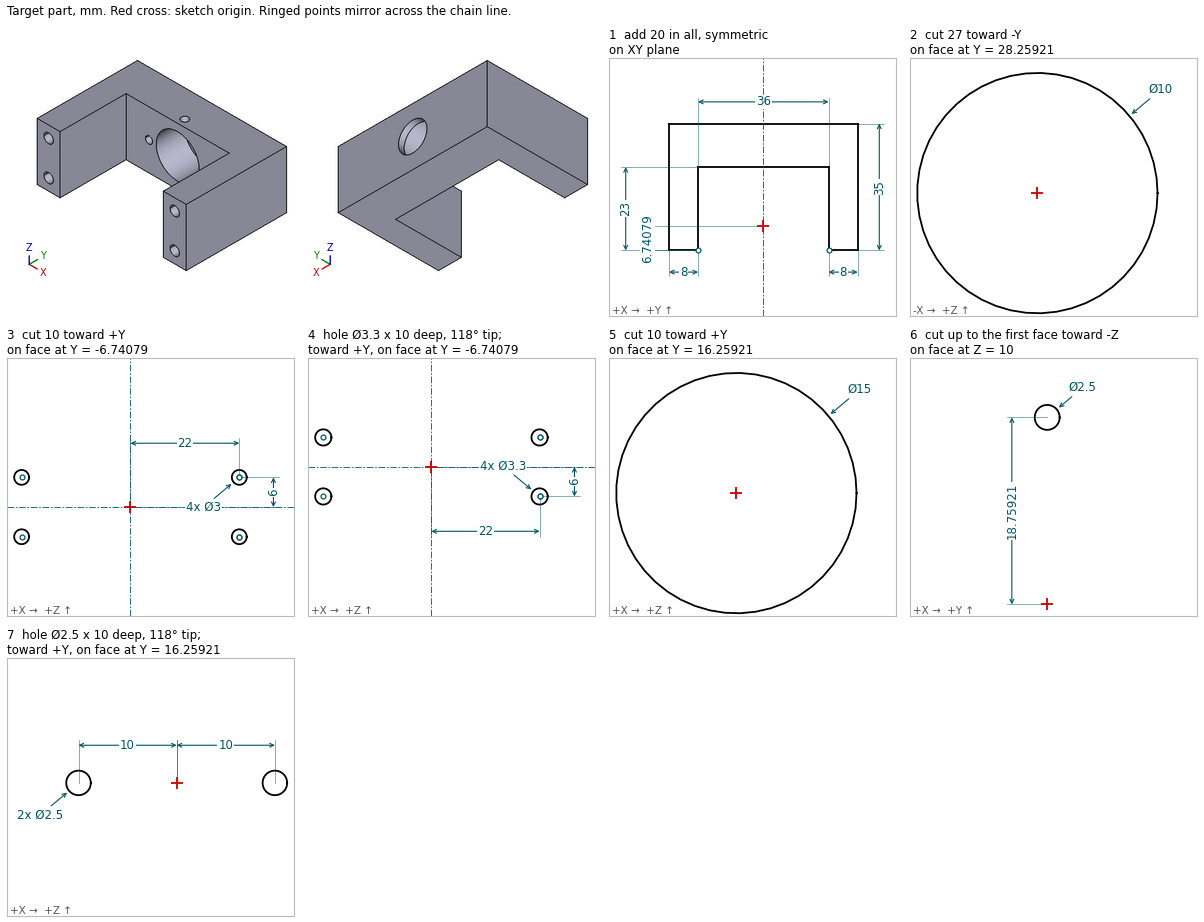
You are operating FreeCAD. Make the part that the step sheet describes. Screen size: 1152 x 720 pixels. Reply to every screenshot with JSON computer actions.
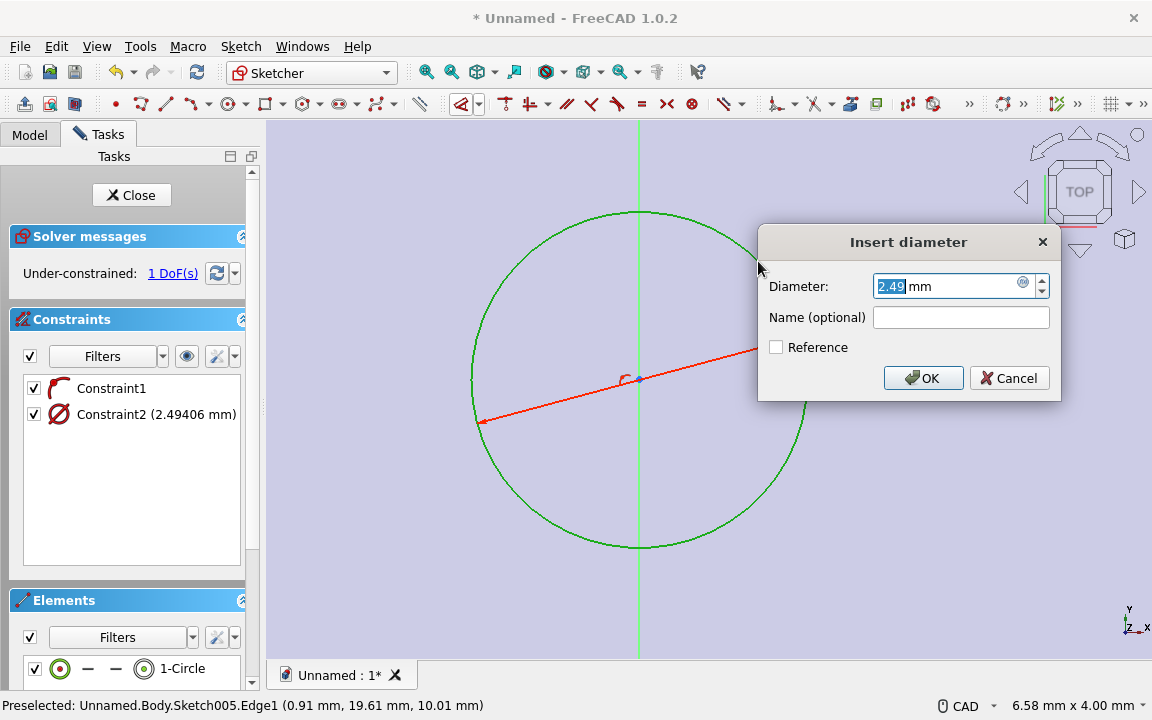
{"action": "type", "text": "2.5"}
{"action": "key", "text": "Return"}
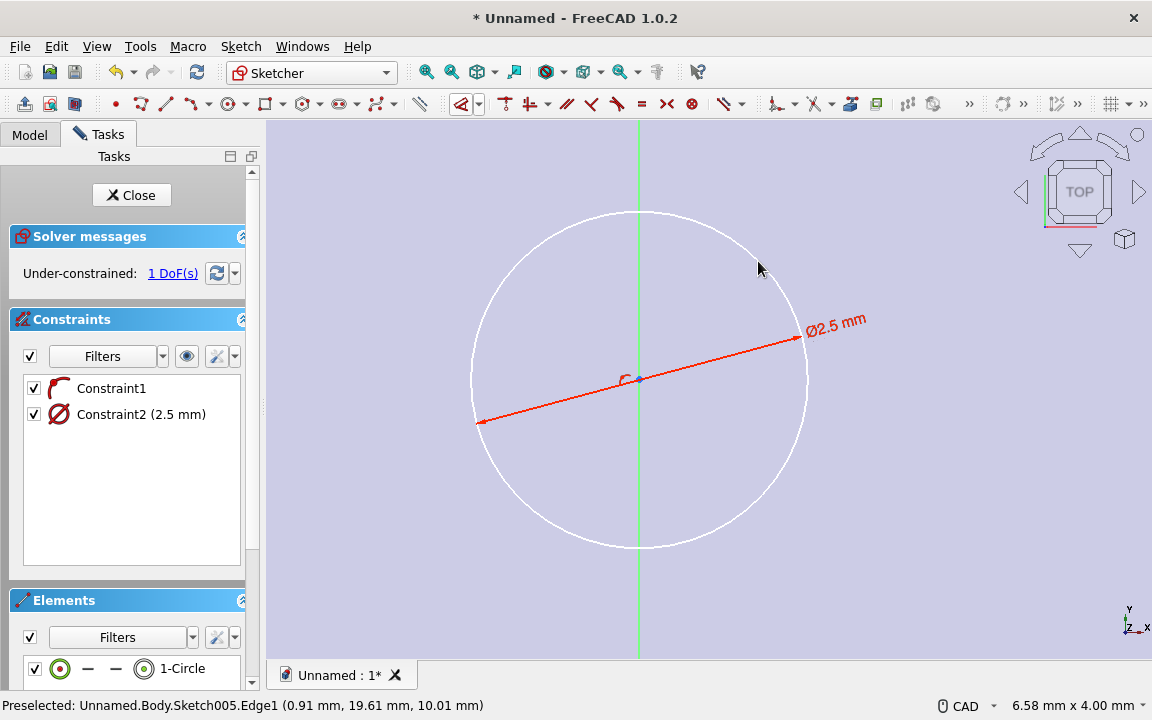
{"action": "left_click", "coordinate": [639, 380]}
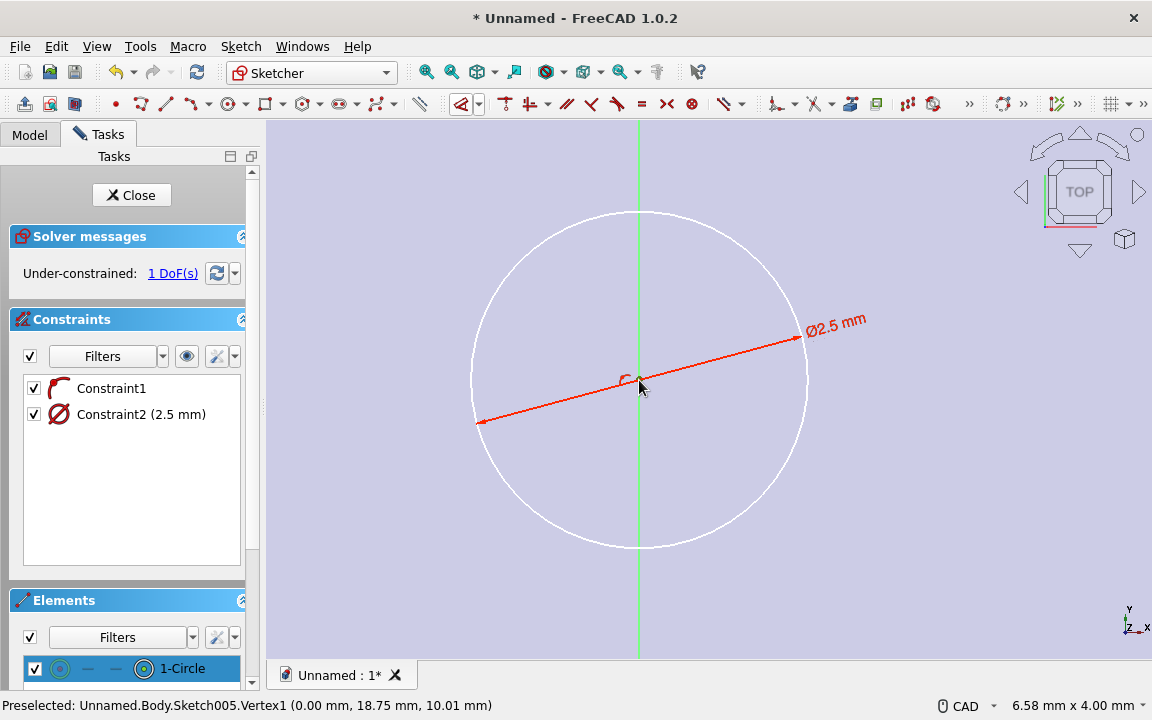
{"action": "left_click", "coordinate": [478, 104]}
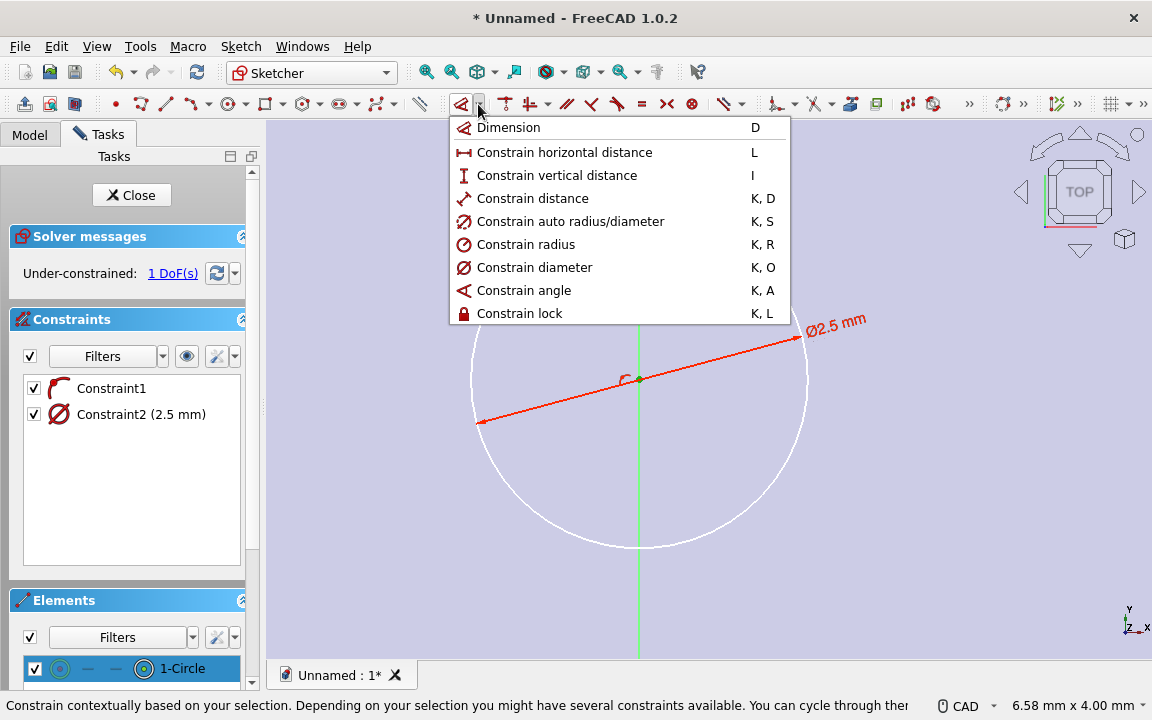
{"action": "left_click", "coordinate": [620, 176]}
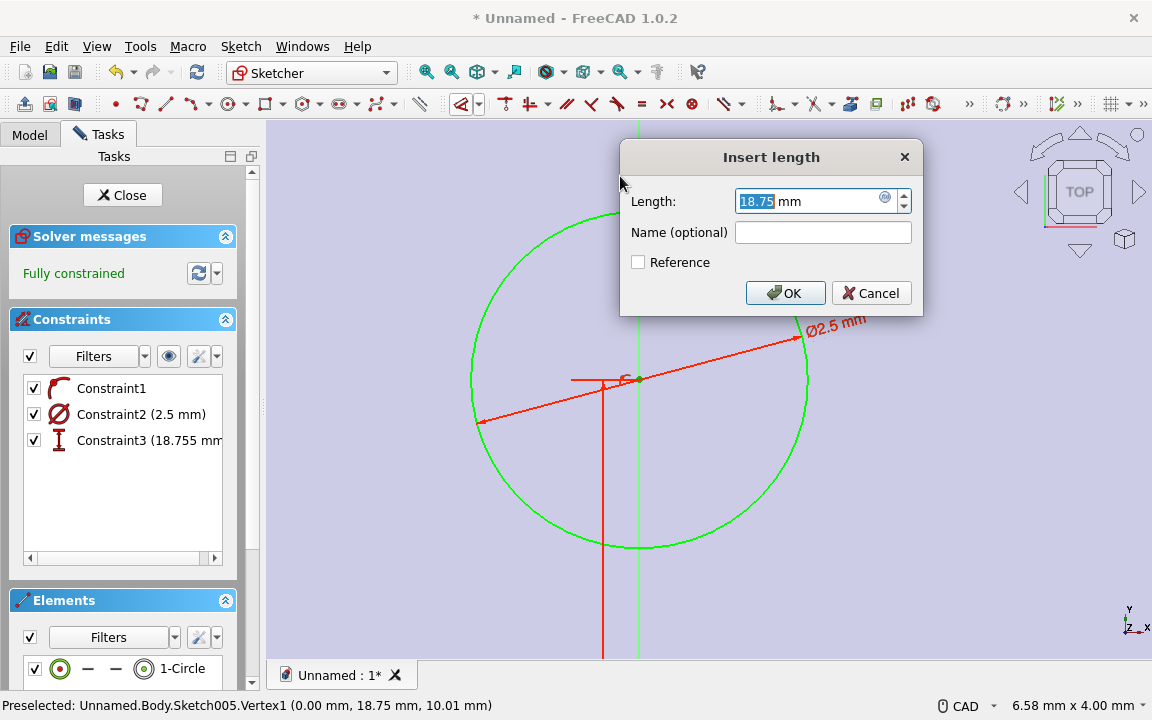
{"action": "type", "text": "18.75921"}
{"action": "key", "text": "Return"}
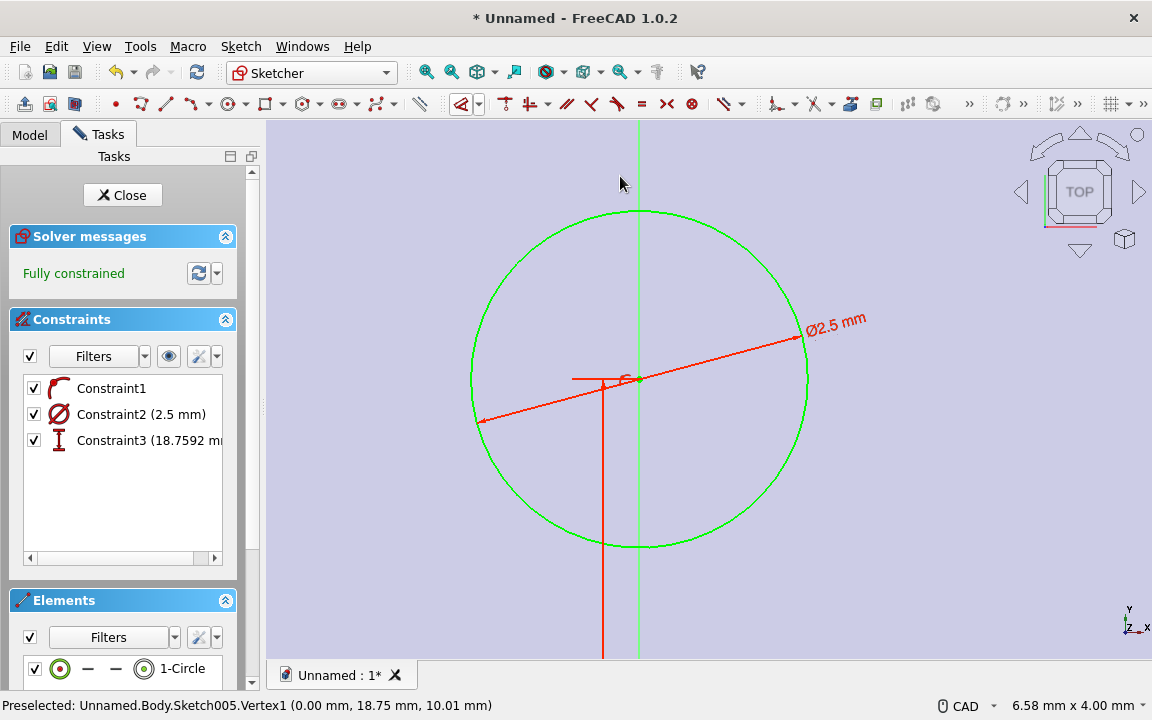
{"action": "left_click", "coordinate": [123, 195]}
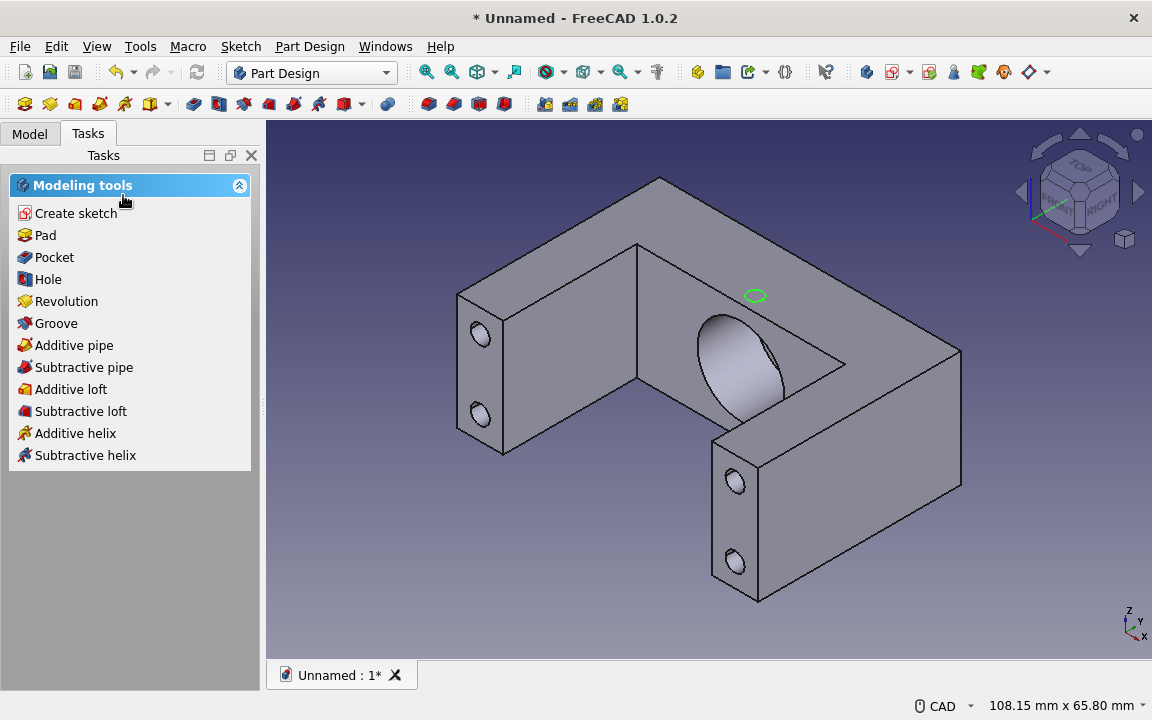
{"action": "left_click", "coordinate": [194, 104]}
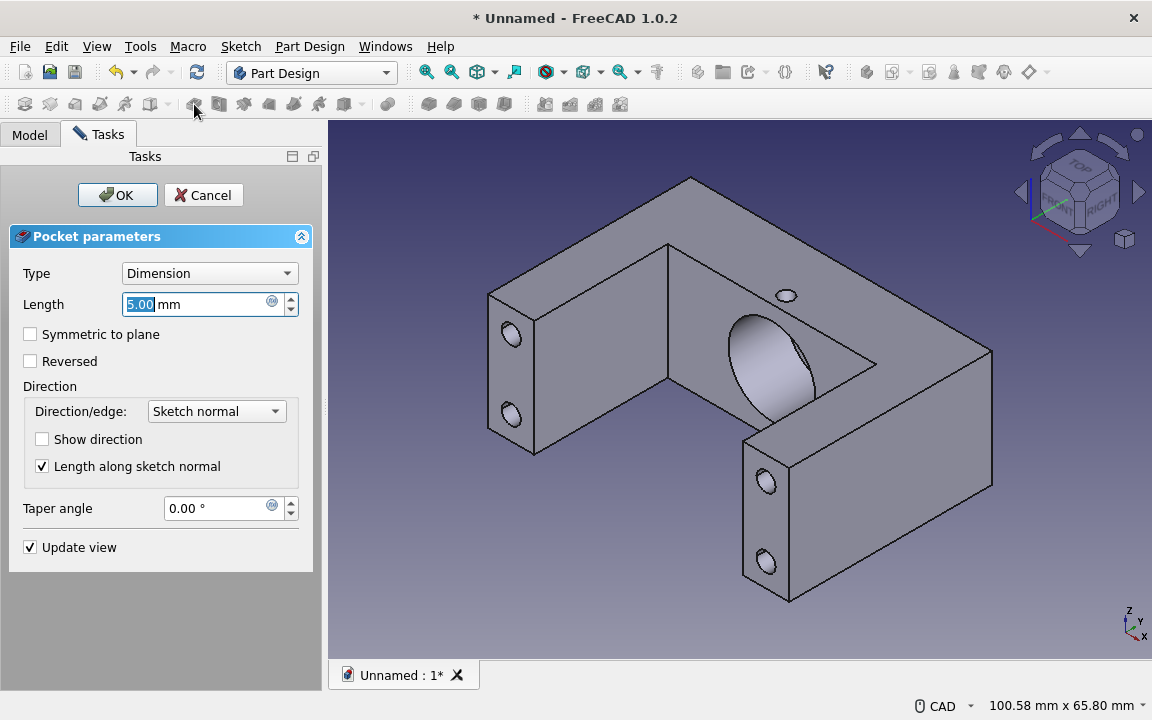
{"action": "left_click", "coordinate": [210, 274]}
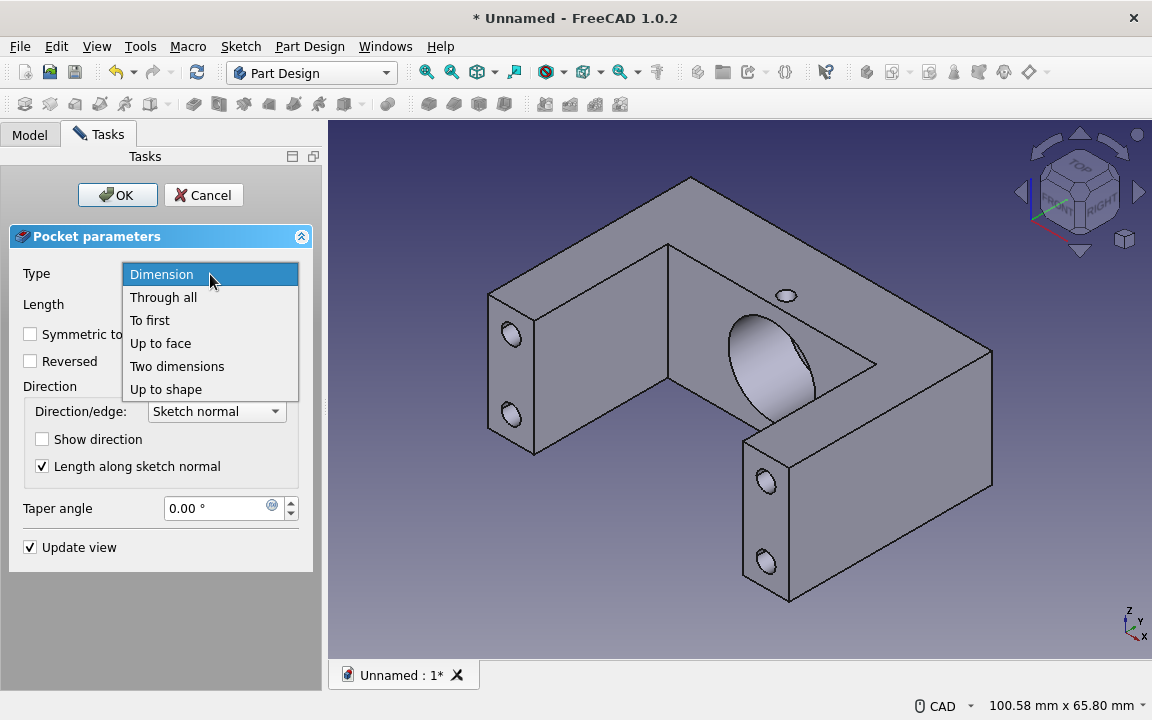
{"action": "left_click", "coordinate": [208, 320]}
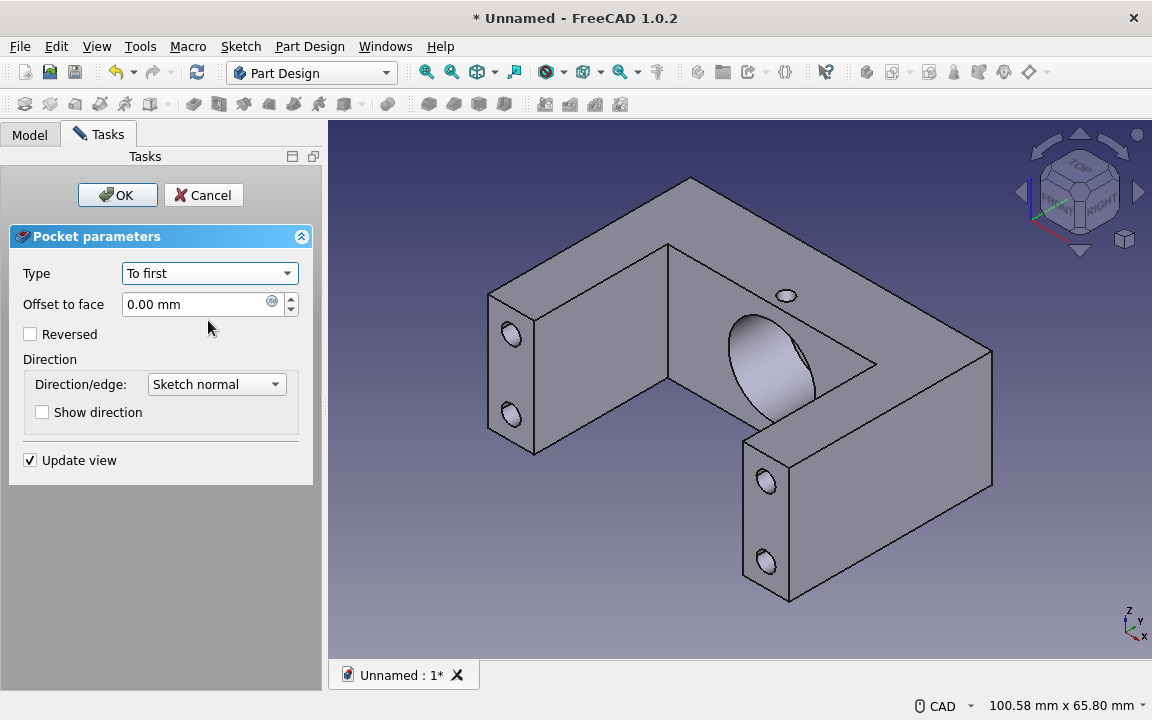
{"action": "left_click", "coordinate": [118, 195]}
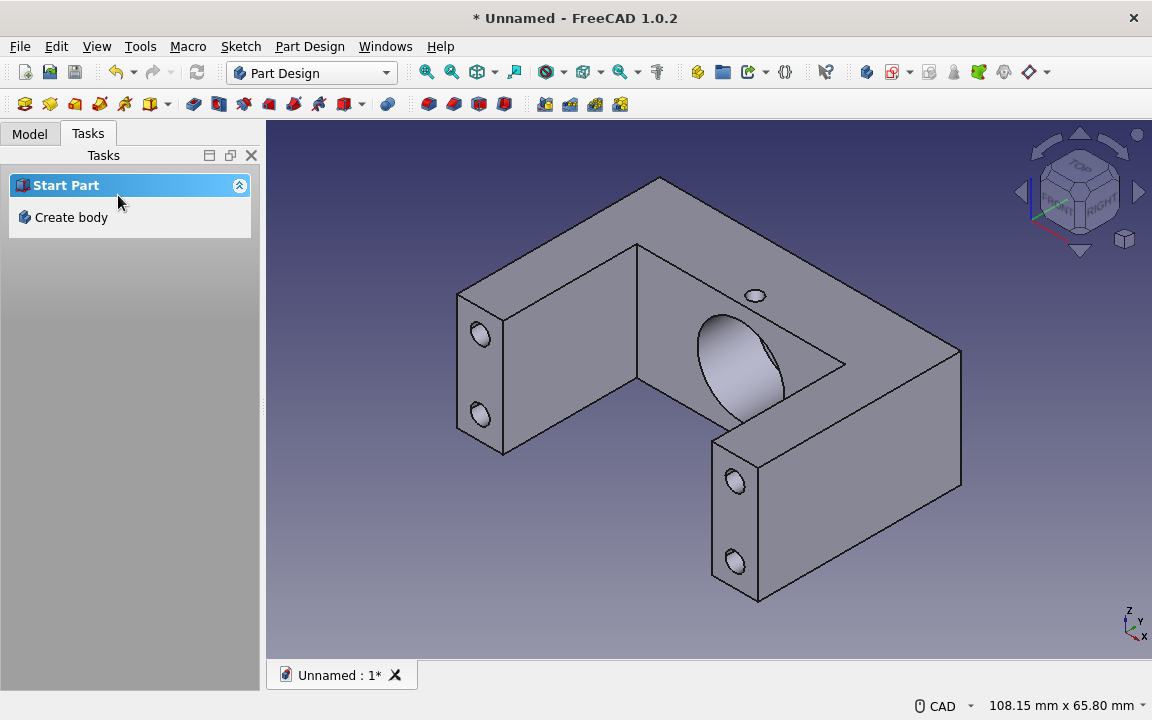
{"action": "left_click", "coordinate": [800, 366]}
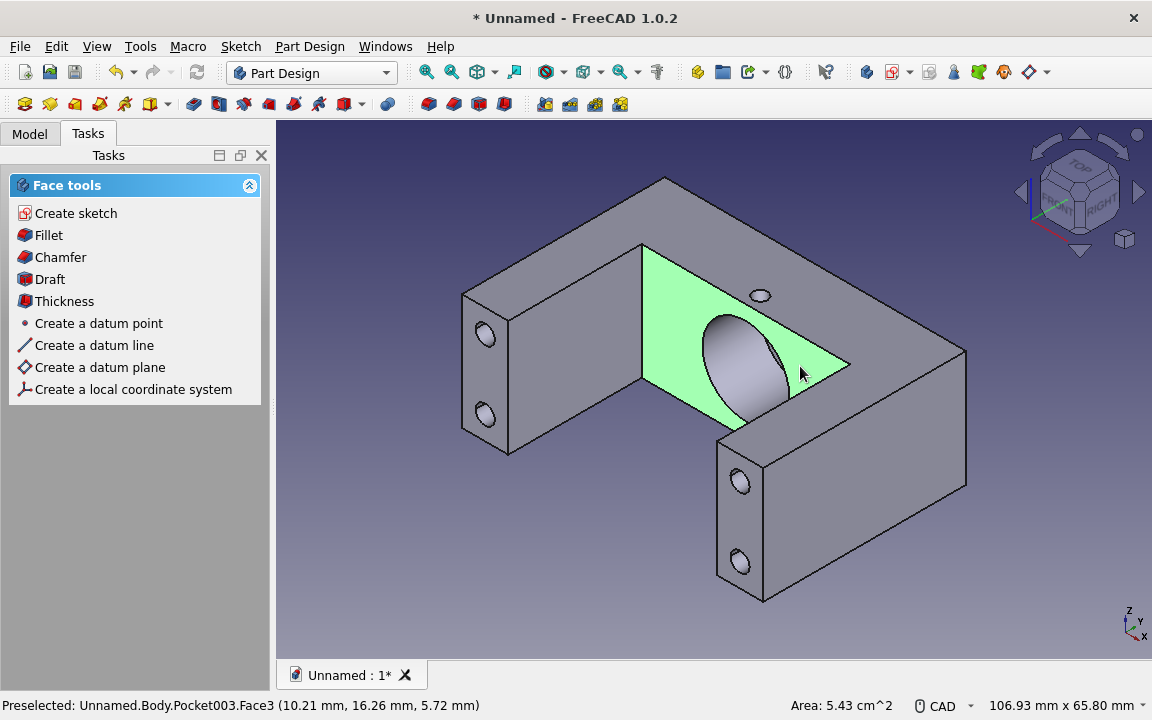
{"action": "left_click", "coordinate": [892, 72]}